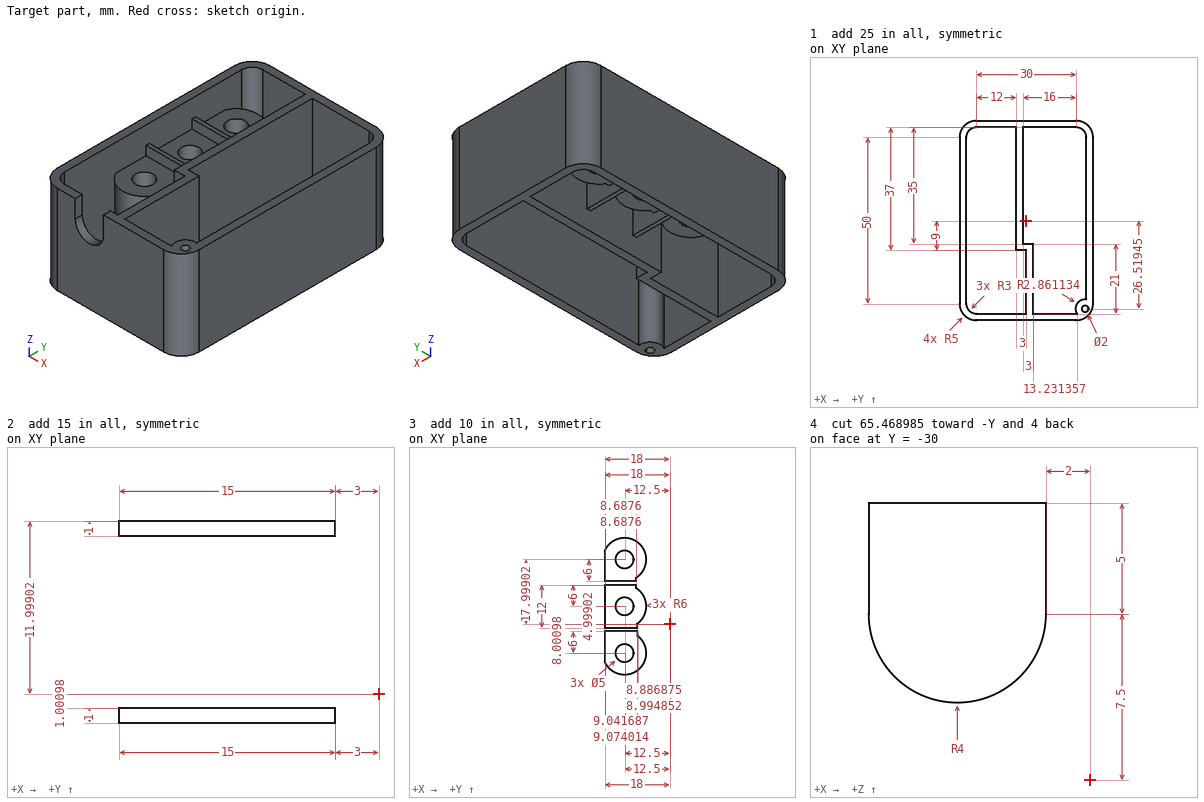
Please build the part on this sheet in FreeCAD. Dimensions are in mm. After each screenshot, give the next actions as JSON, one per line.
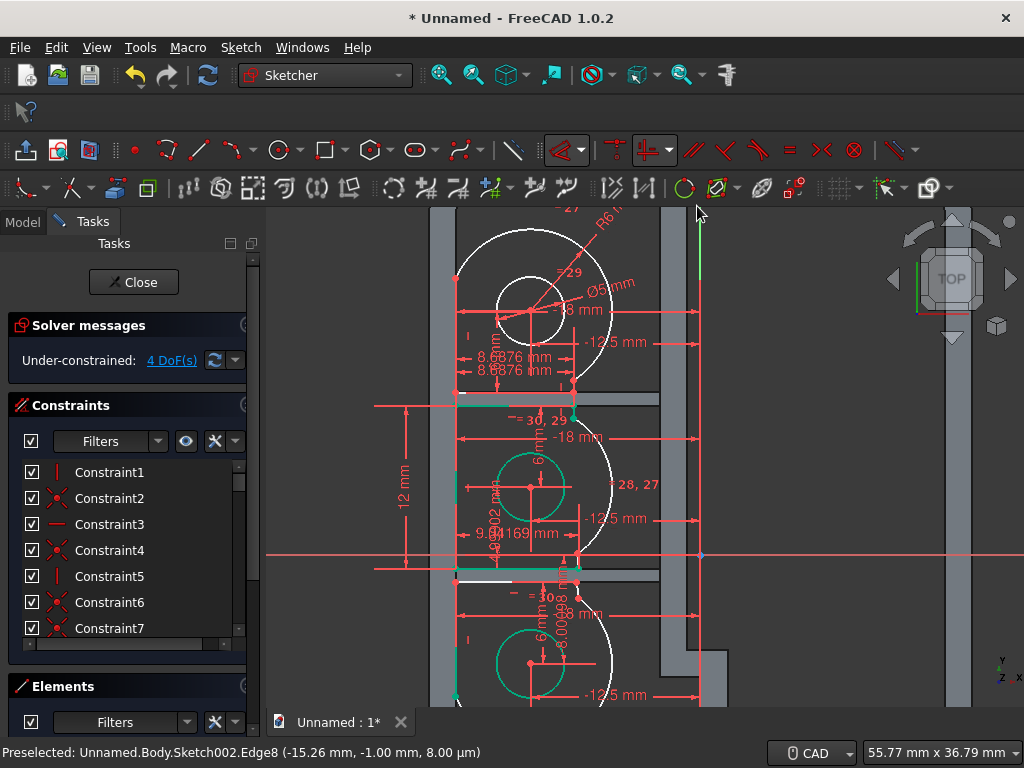
{"action": "left_click", "coordinate": [540, 582]}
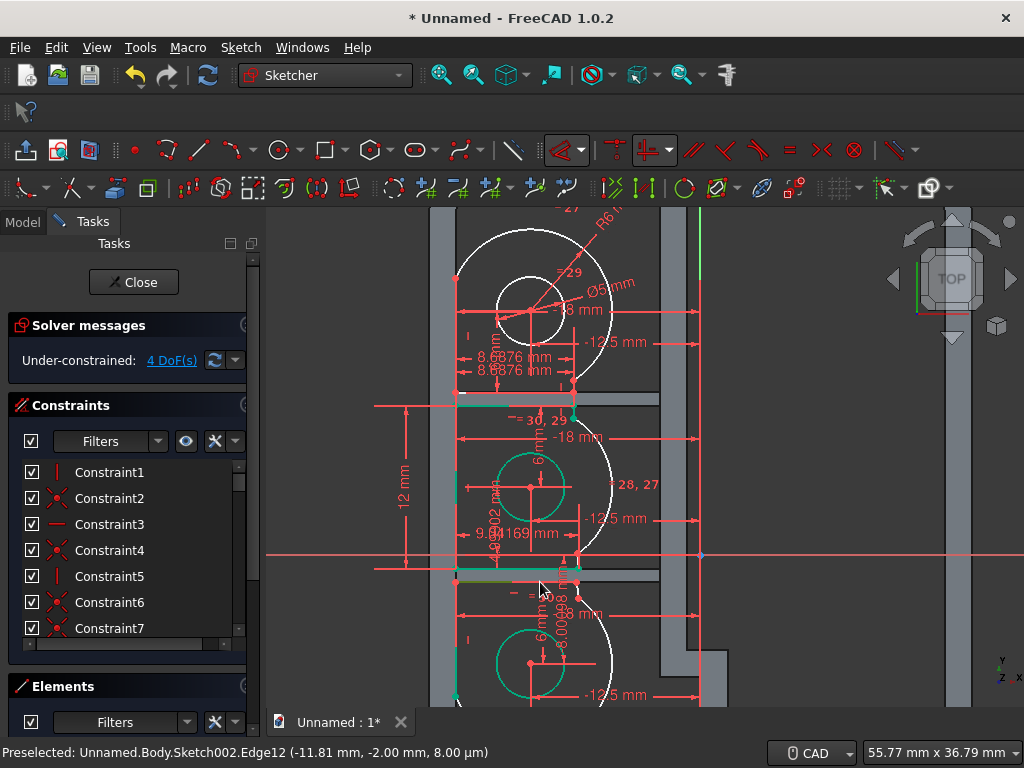
{"action": "key", "text": "l"}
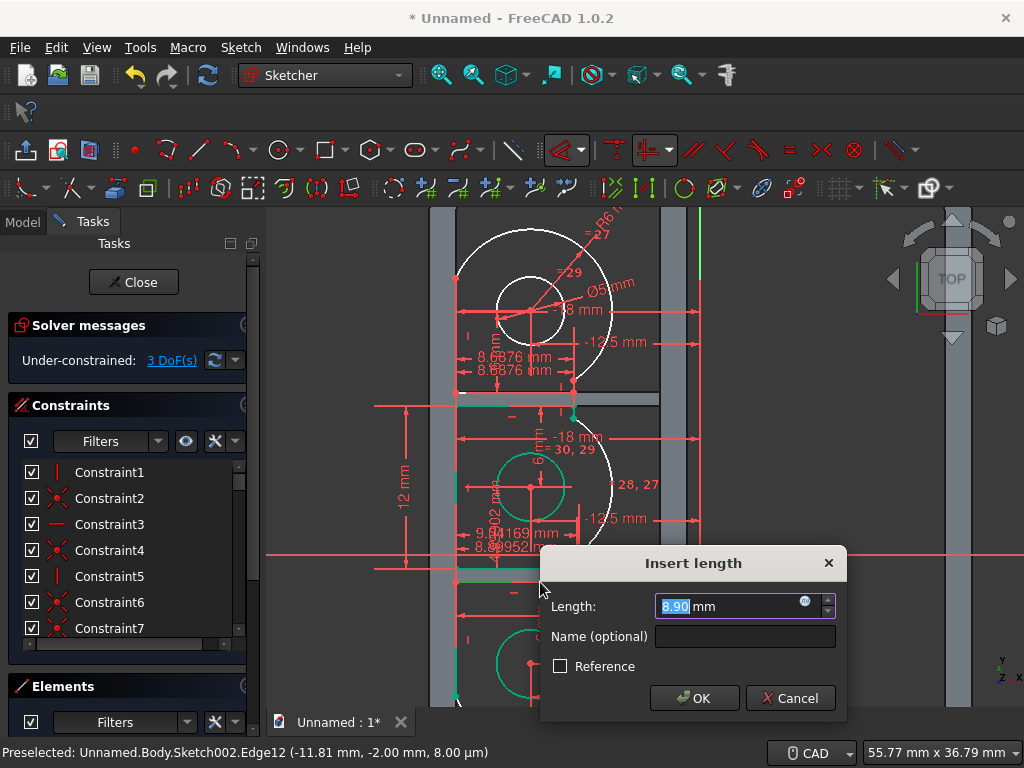
{"action": "type", "text": "9.074014"}
{"action": "key", "text": "Return"}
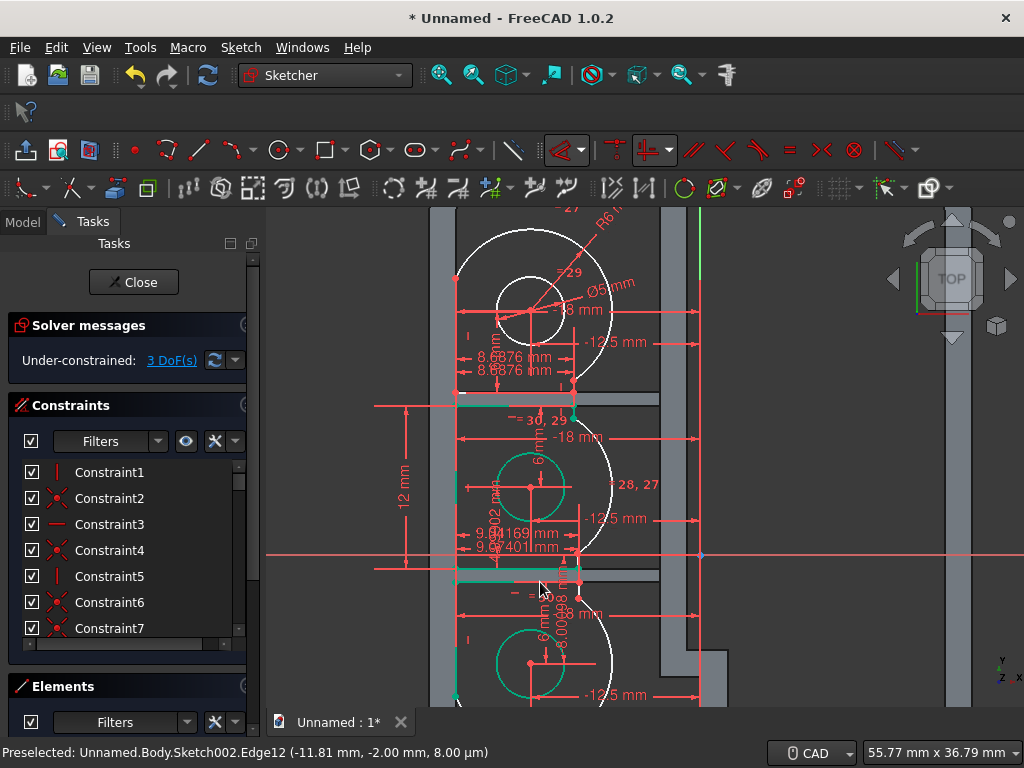
{"action": "left_click", "coordinate": [531, 311]}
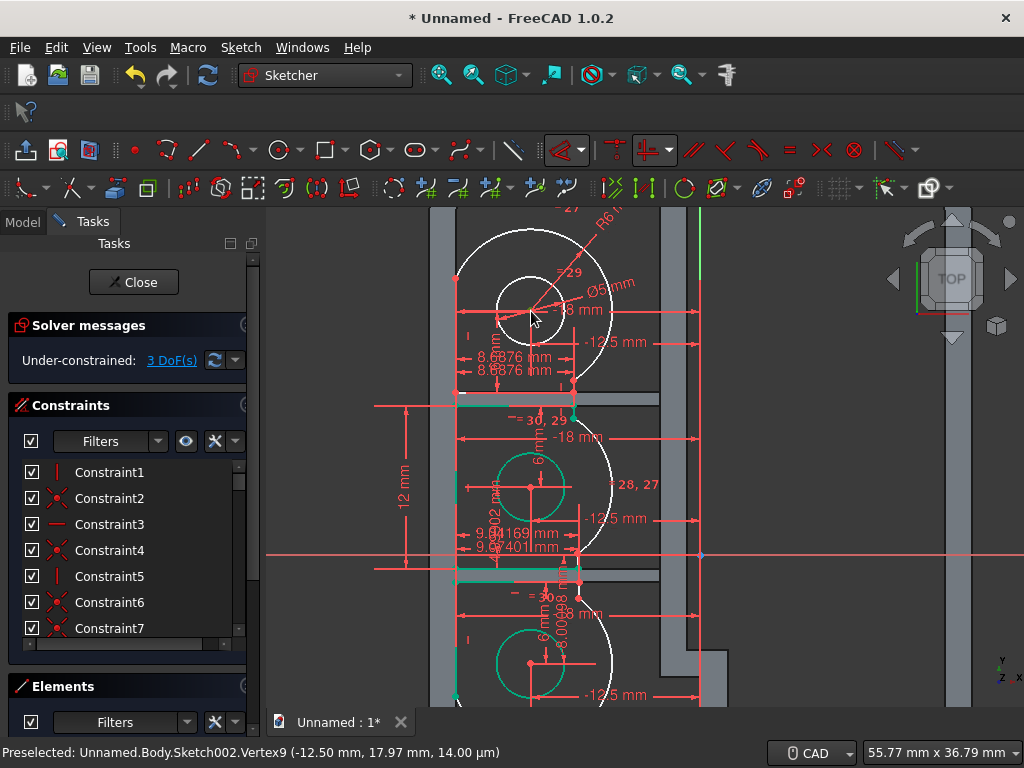
{"action": "left_click", "coordinate": [584, 150]}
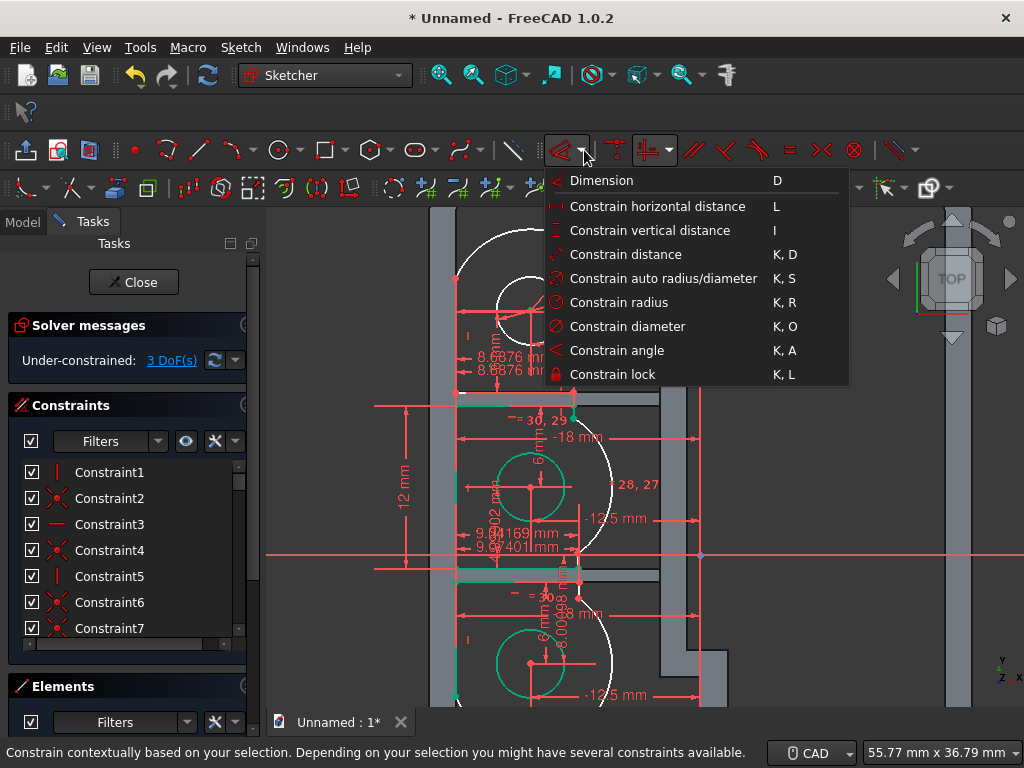
{"action": "left_click", "coordinate": [697, 230]}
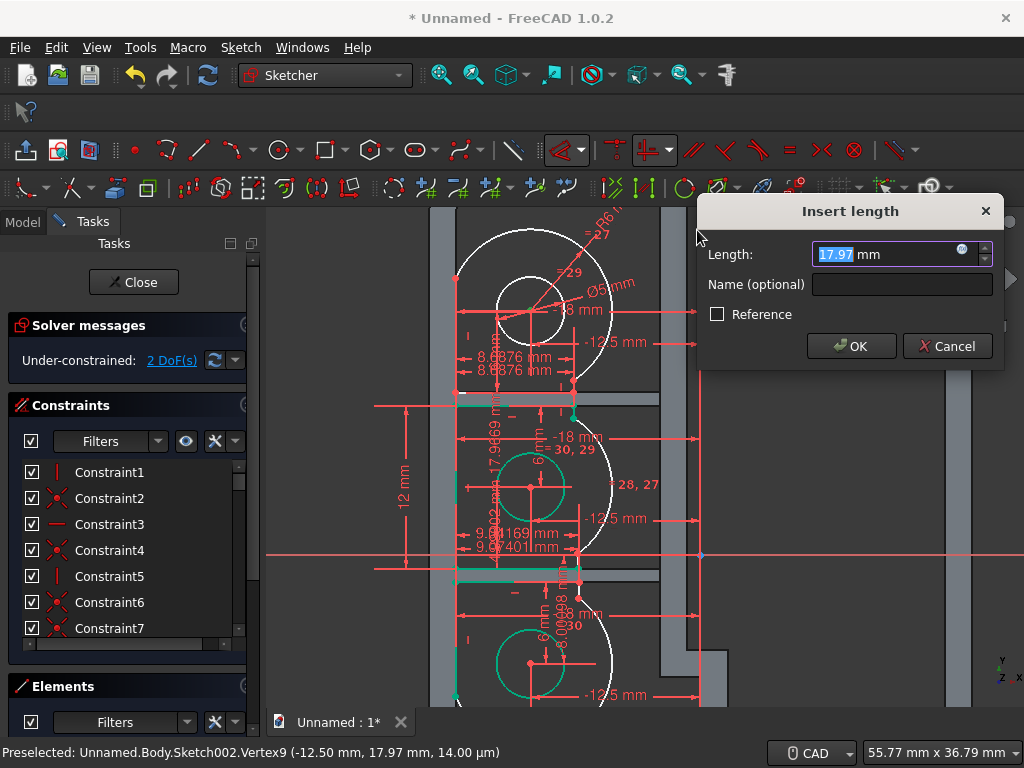
{"action": "type", "text": "17.99902"}
{"action": "key", "text": "Return"}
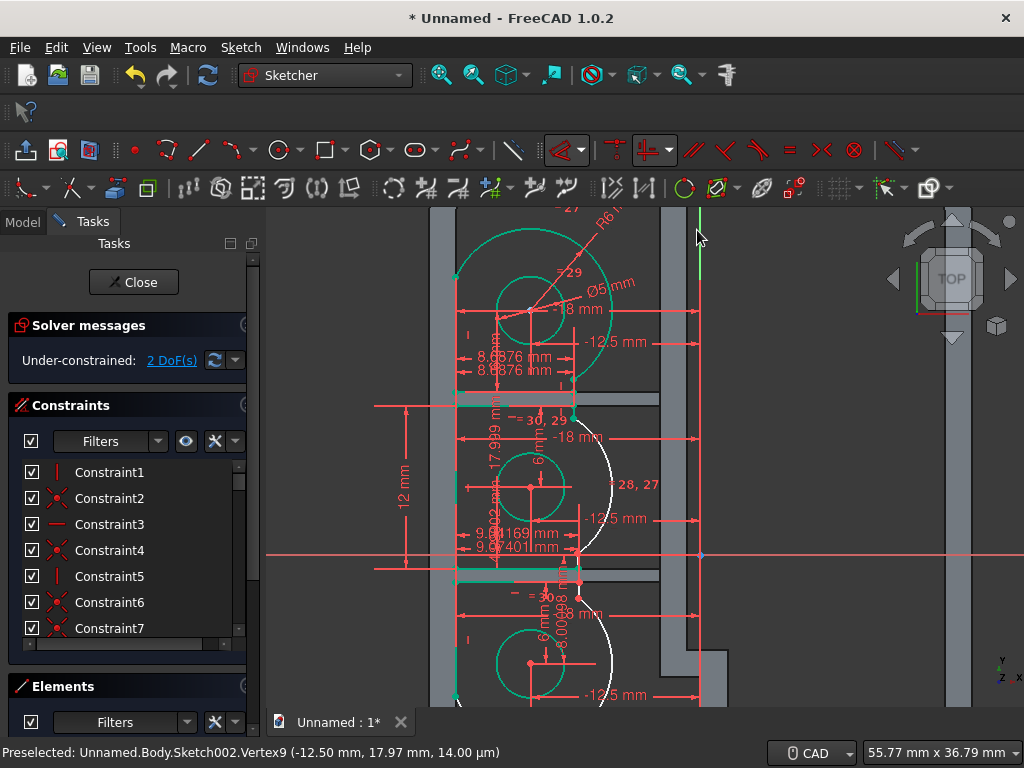
{"action": "left_click", "coordinate": [578, 554]}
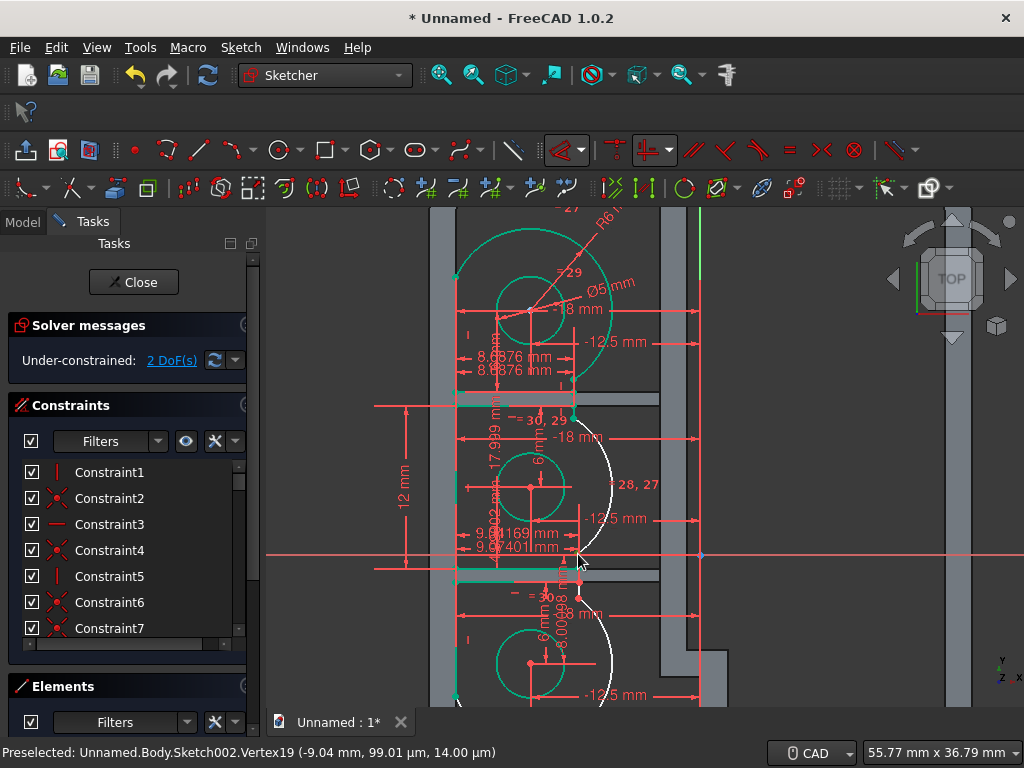
{"action": "key", "text": "l"}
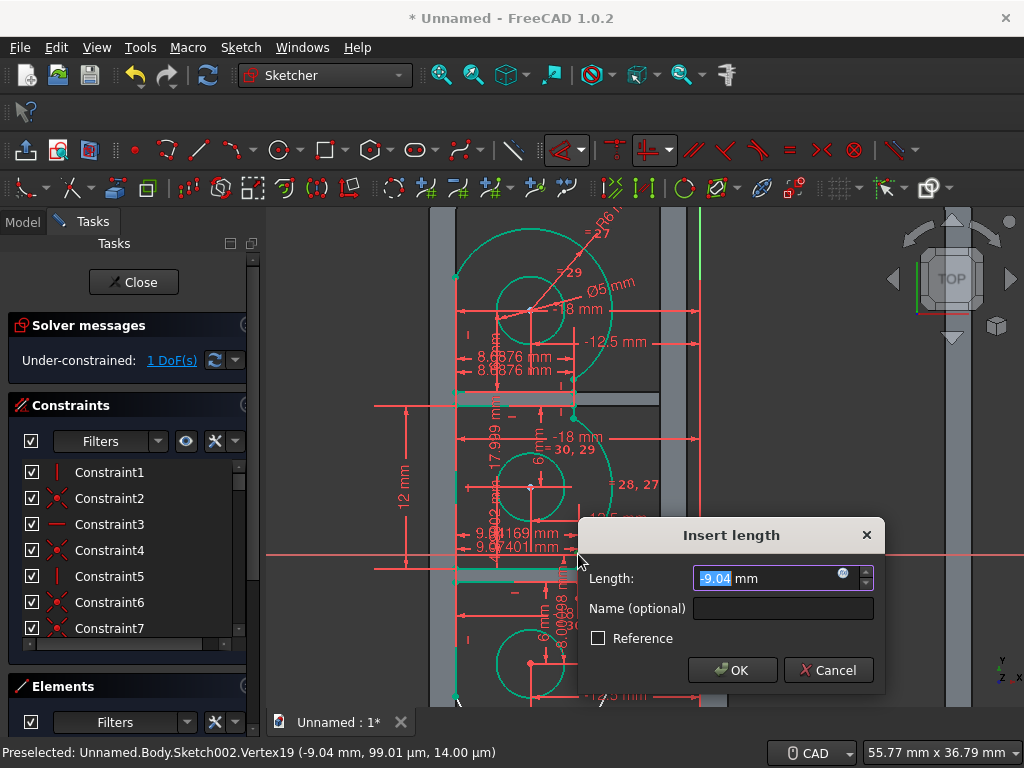
{"action": "type", "text": "-8.994852"}
{"action": "key", "text": "Return"}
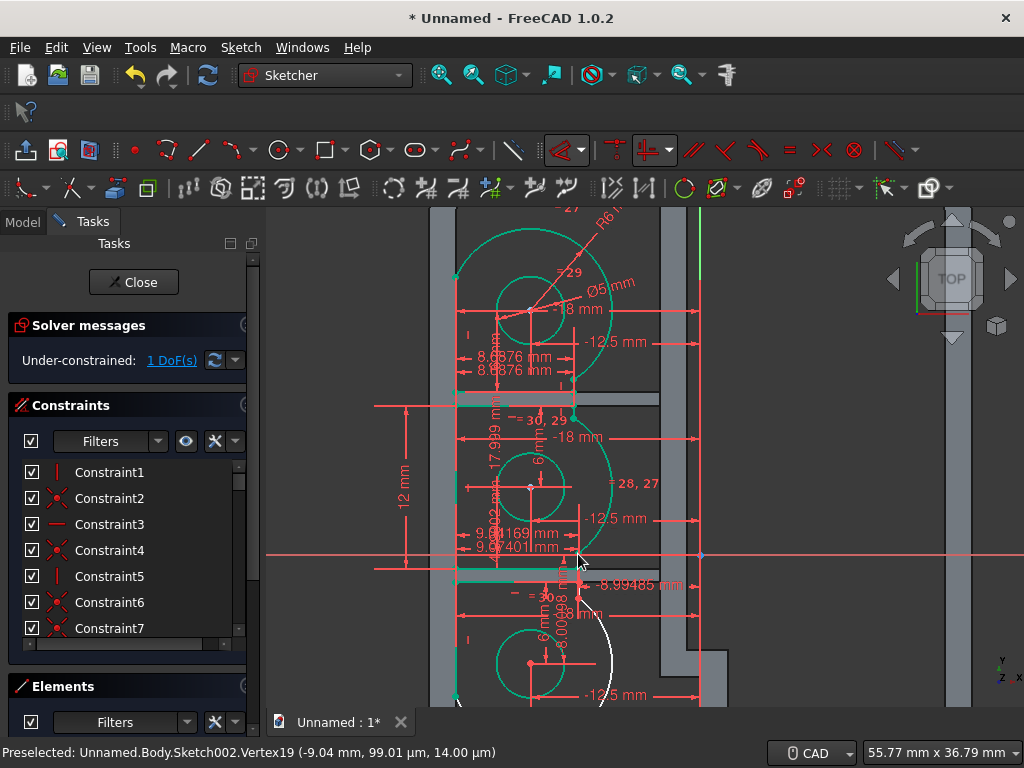
{"action": "left_click", "coordinate": [579, 598]}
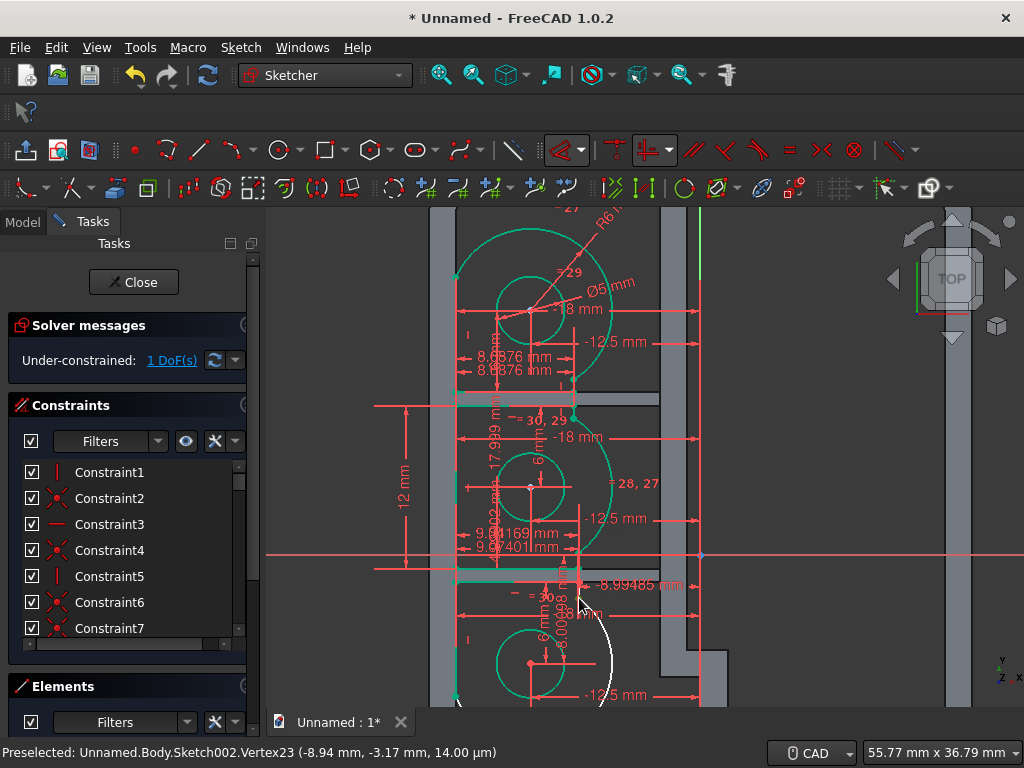
{"action": "left_click", "coordinate": [584, 150]}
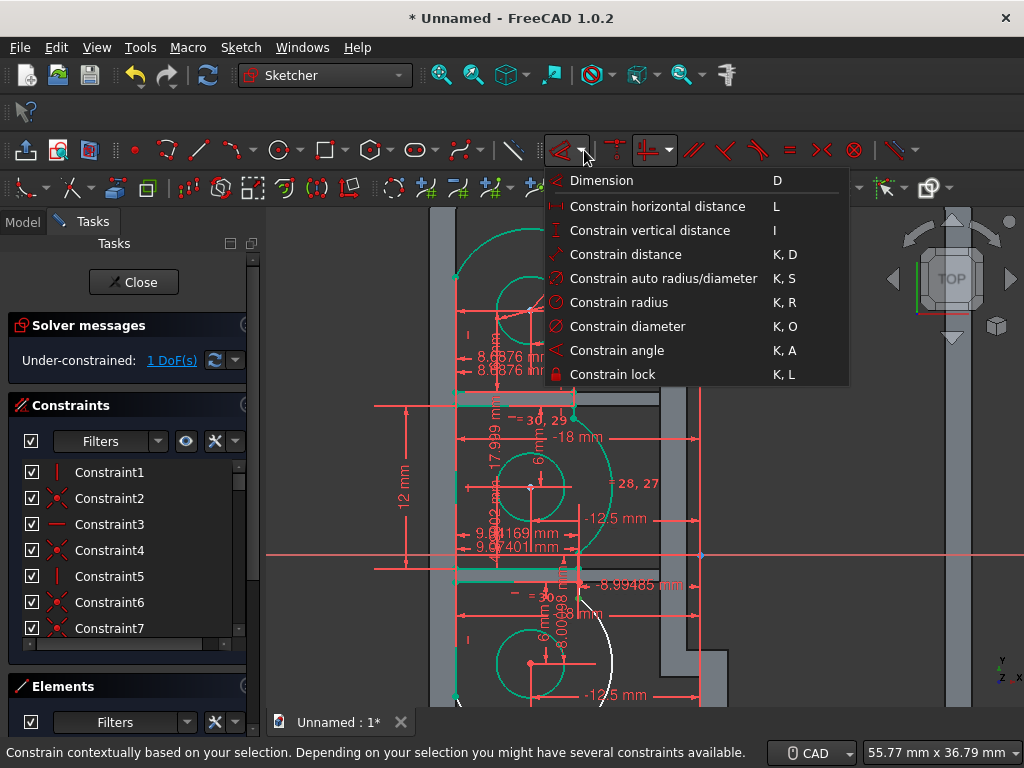
{"action": "left_click", "coordinate": [697, 206]}